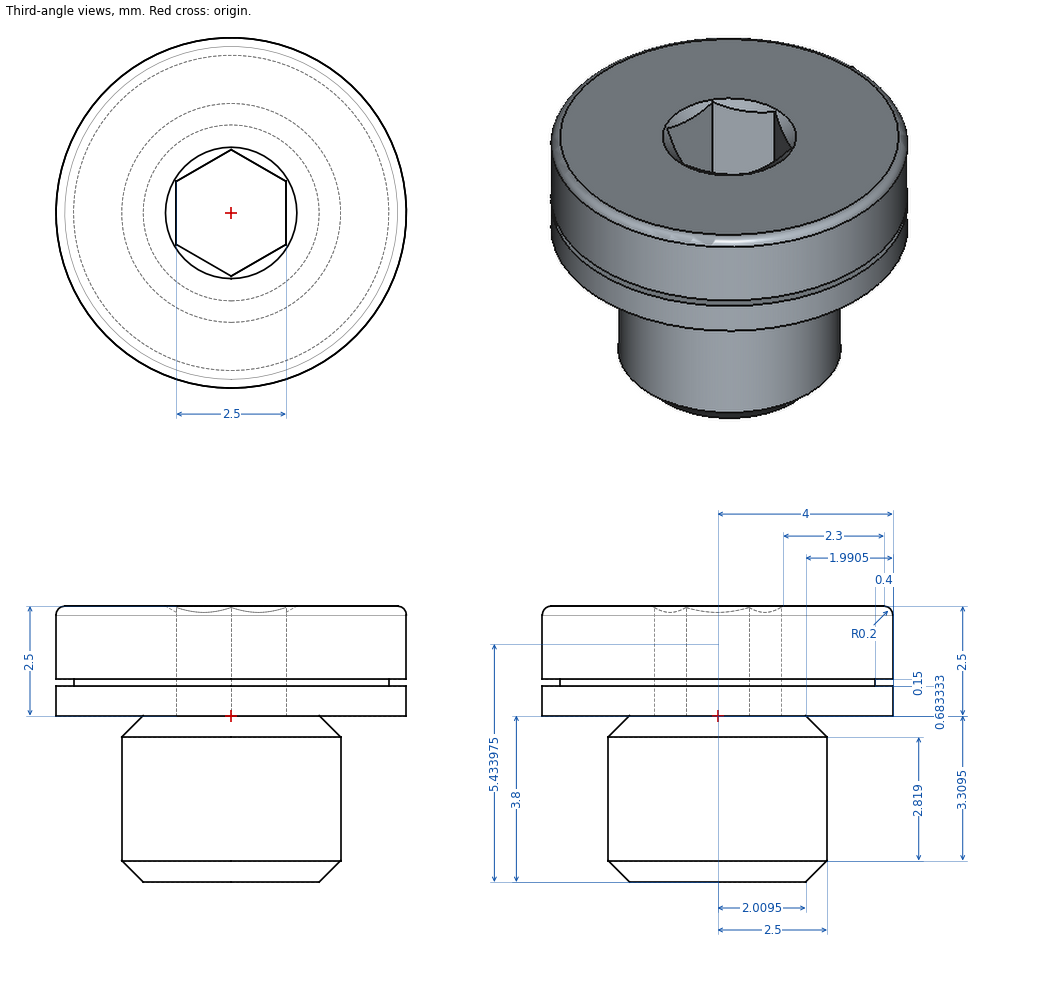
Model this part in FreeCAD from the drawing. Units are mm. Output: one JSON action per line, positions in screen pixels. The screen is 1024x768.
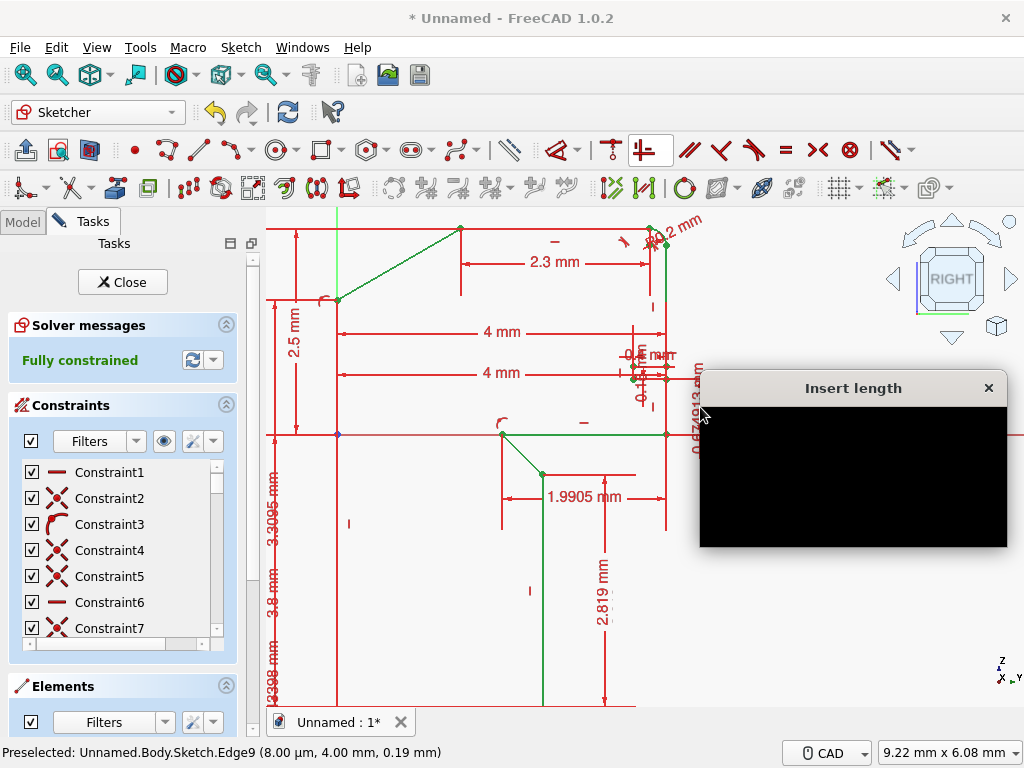
{"action": "type", "text": "0.683333"}
{"action": "key", "text": "Return"}
{"action": "key", "text": "Escape"}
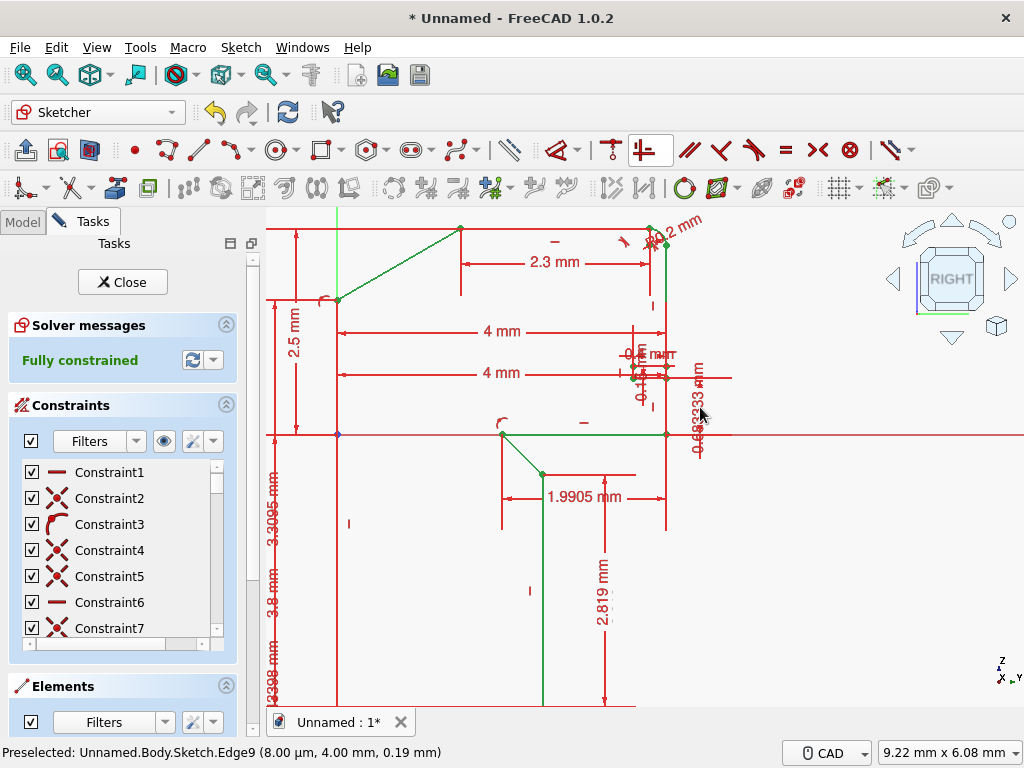
{"action": "left_click", "coordinate": [123, 282]}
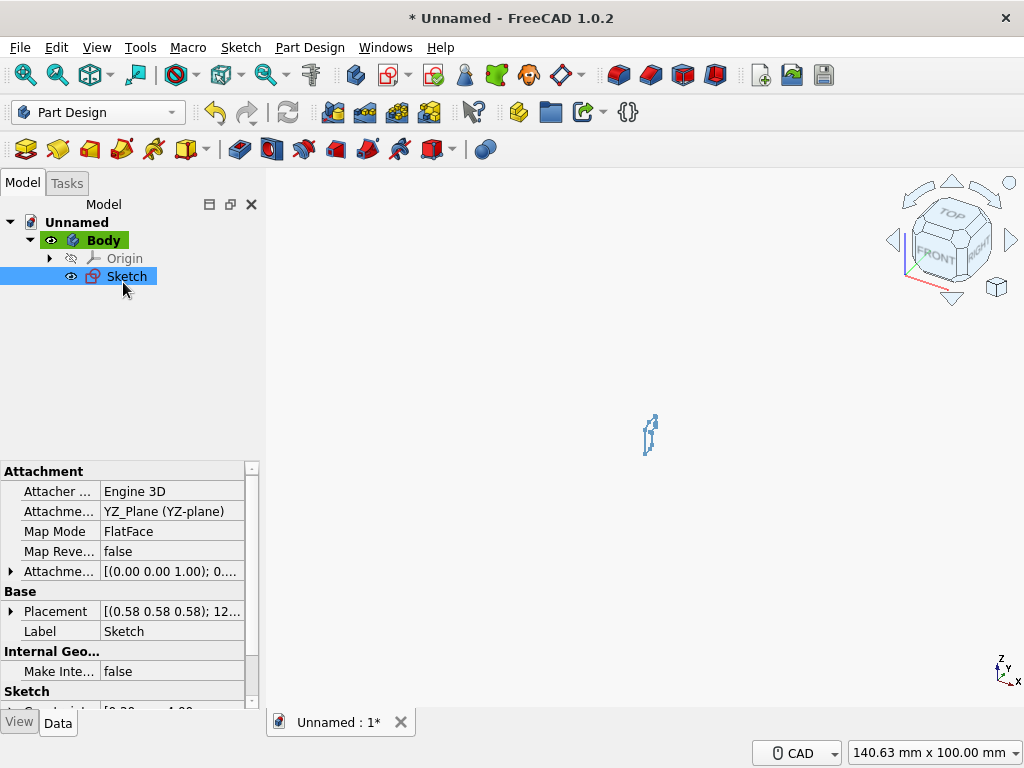
{"action": "left_click", "coordinate": [58, 150]}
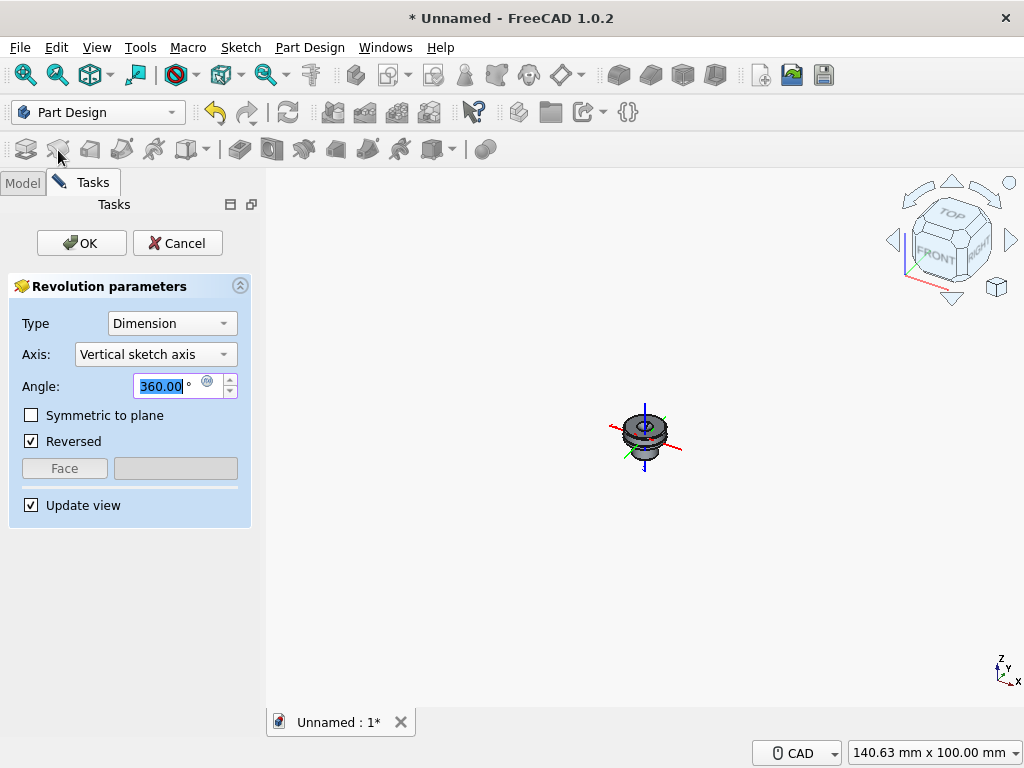
{"action": "left_click", "coordinate": [82, 243]}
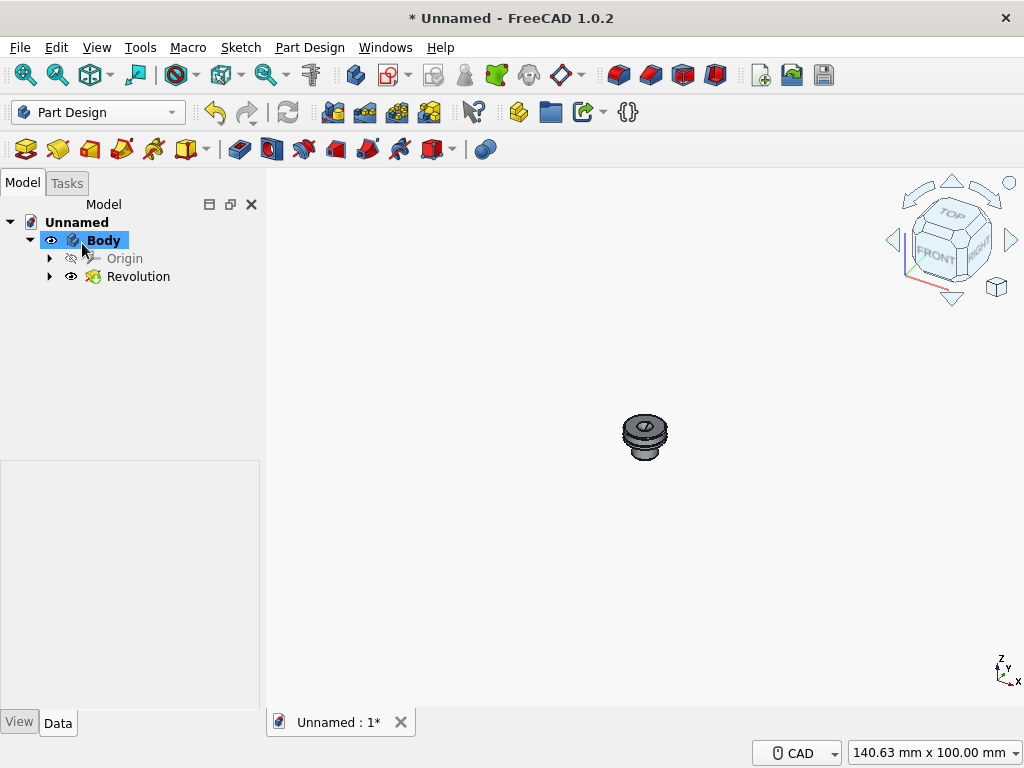
{"action": "left_click", "coordinate": [26, 76]}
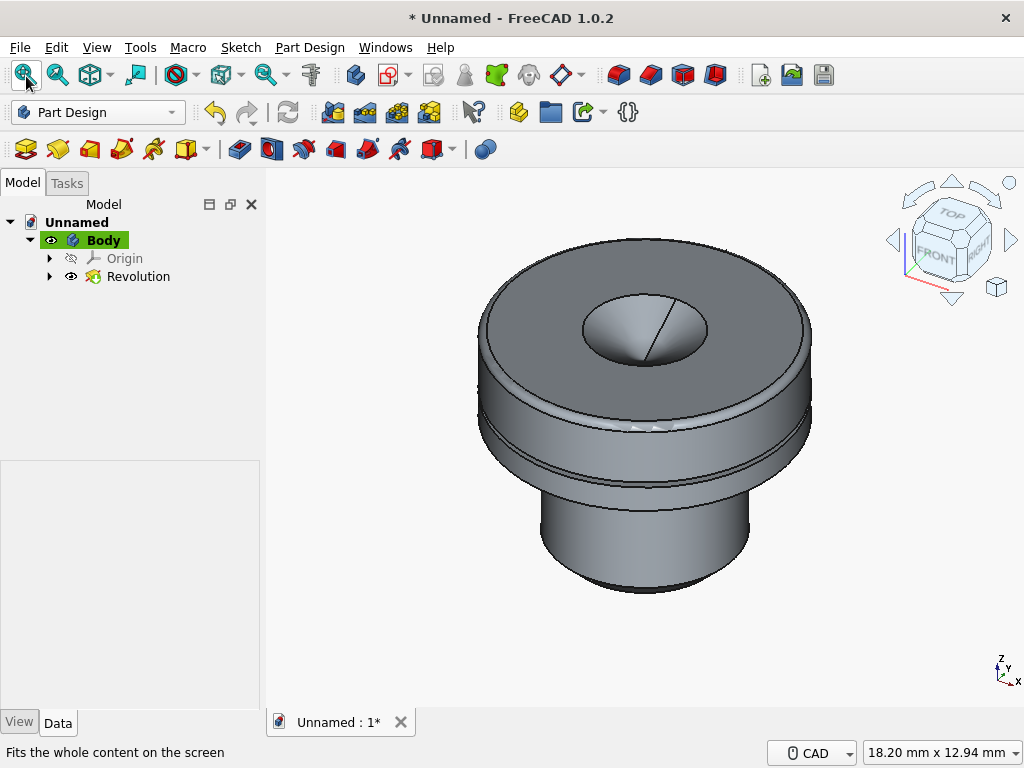
{"action": "left_click", "coordinate": [729, 297]}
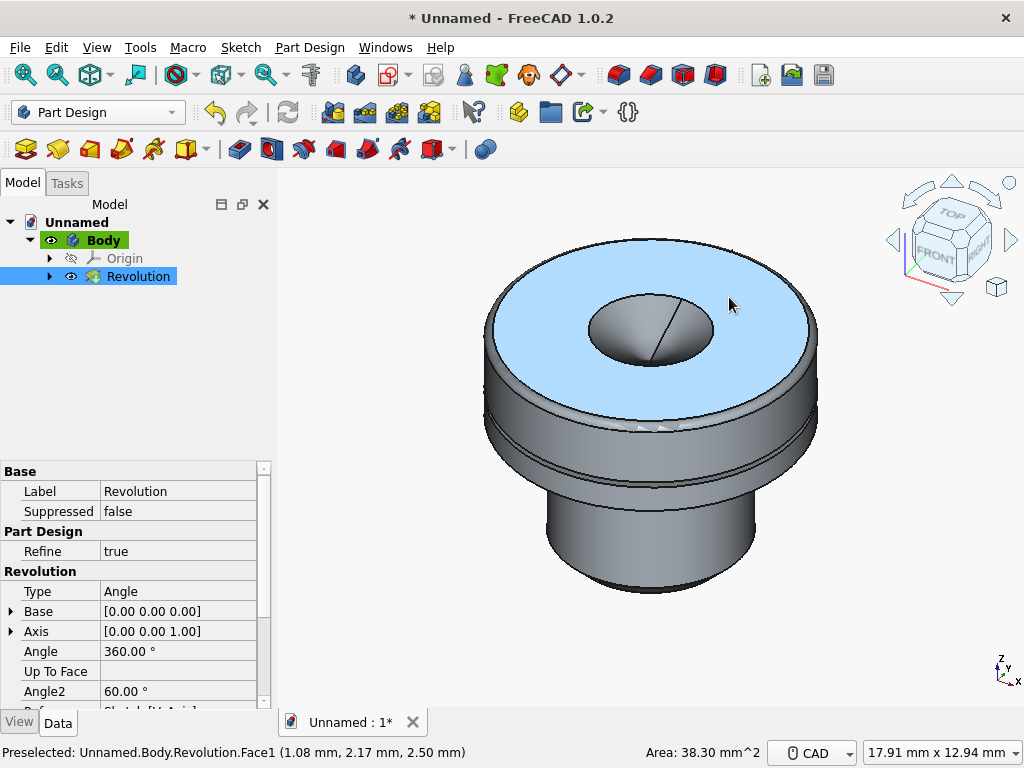
{"action": "left_click", "coordinate": [388, 76]}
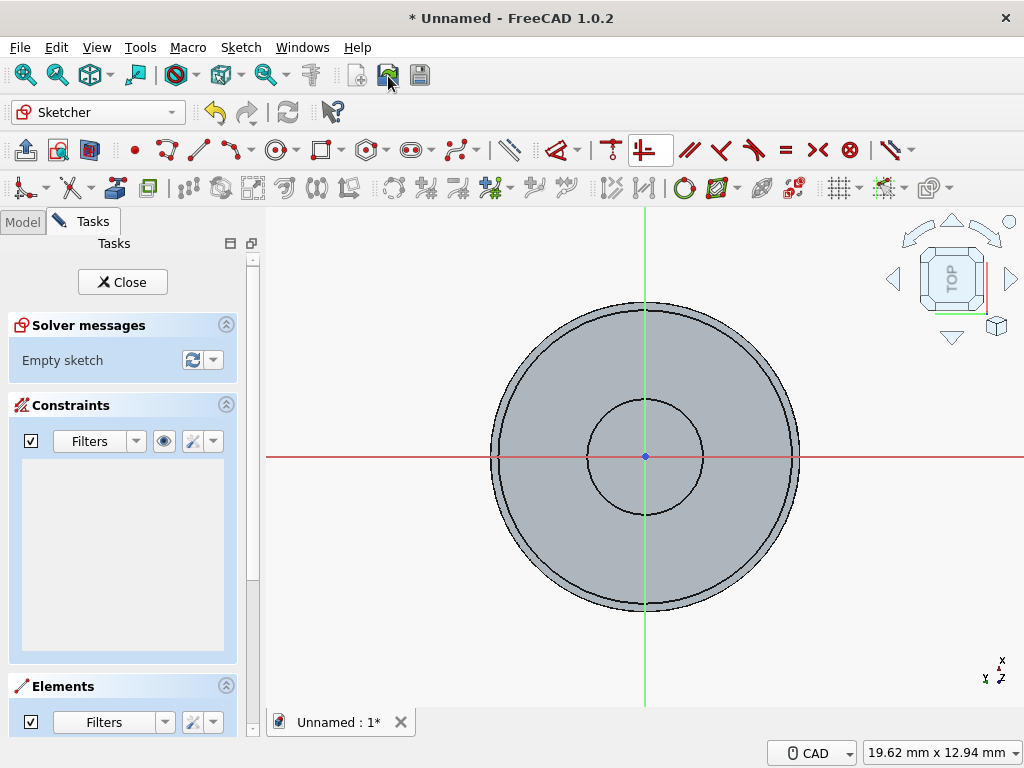
{"action": "scroll", "coordinate": [675, 457], "scroll_direction": "up", "scroll_amount": 6}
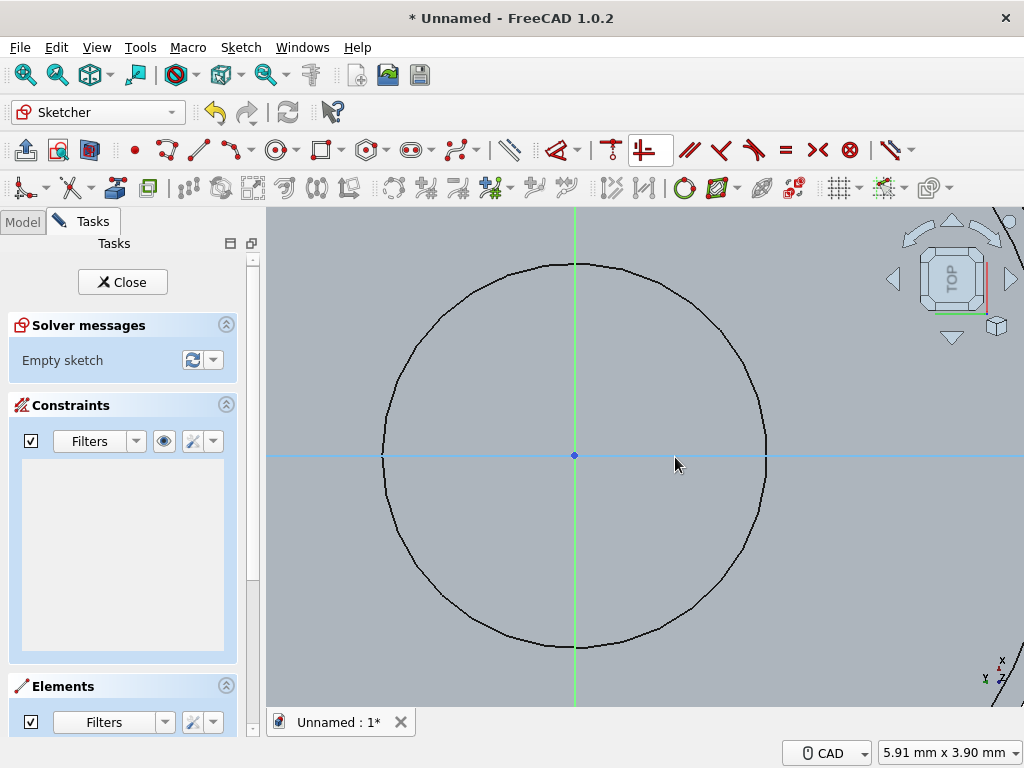
{"action": "key", "text": "g p 6"}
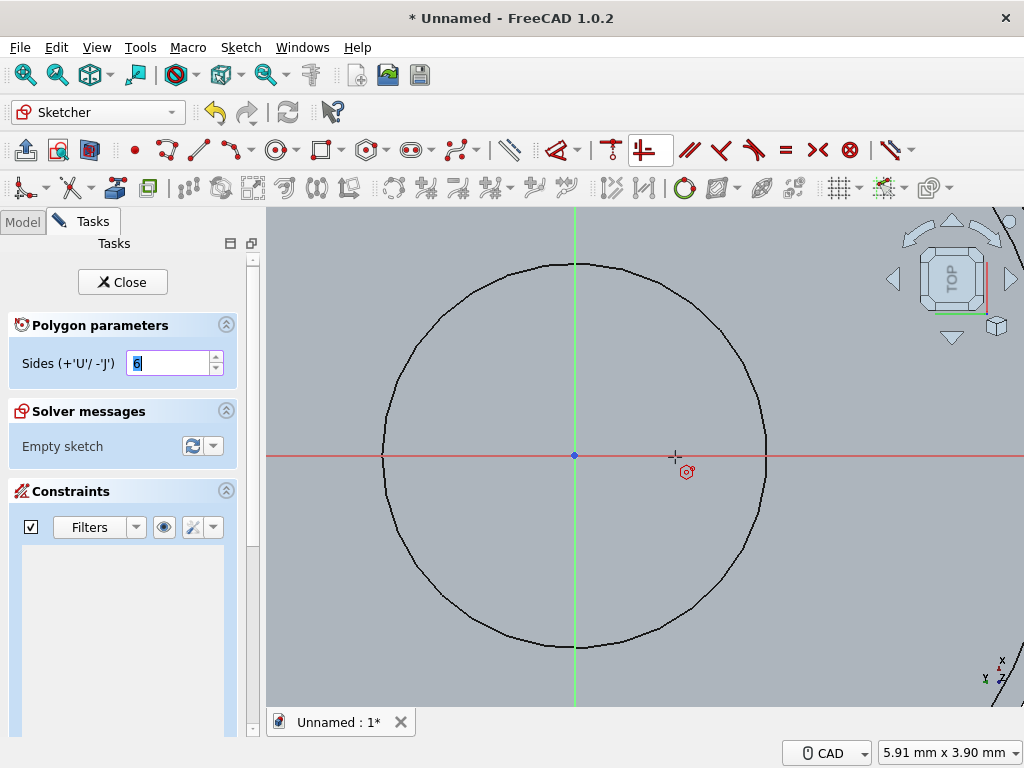
{"action": "left_click", "coordinate": [575, 456]}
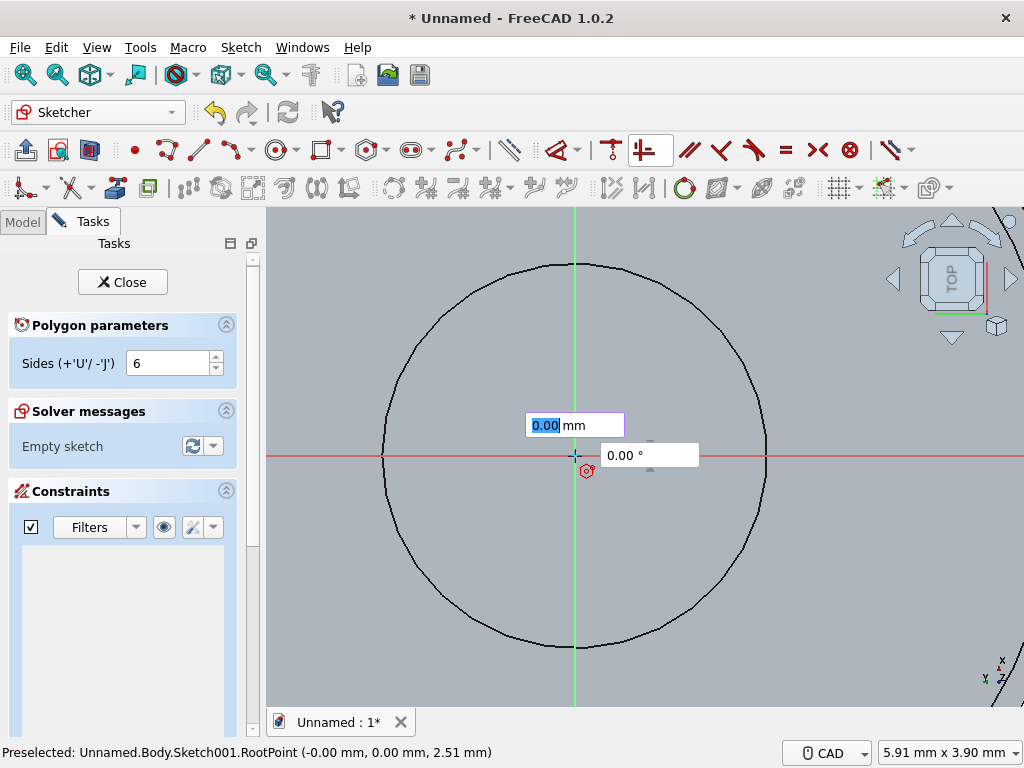
{"action": "left_click", "coordinate": [760, 456]}
{"action": "right_click", "coordinate": [760, 456]}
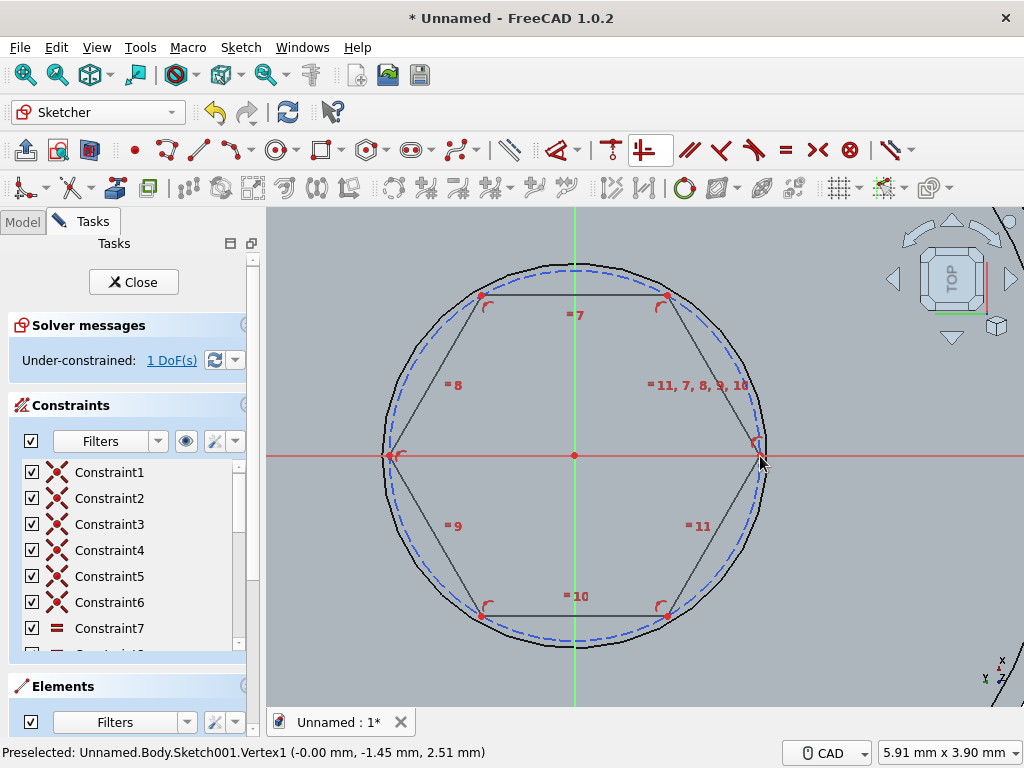
{"action": "left_click", "coordinate": [556, 150]}